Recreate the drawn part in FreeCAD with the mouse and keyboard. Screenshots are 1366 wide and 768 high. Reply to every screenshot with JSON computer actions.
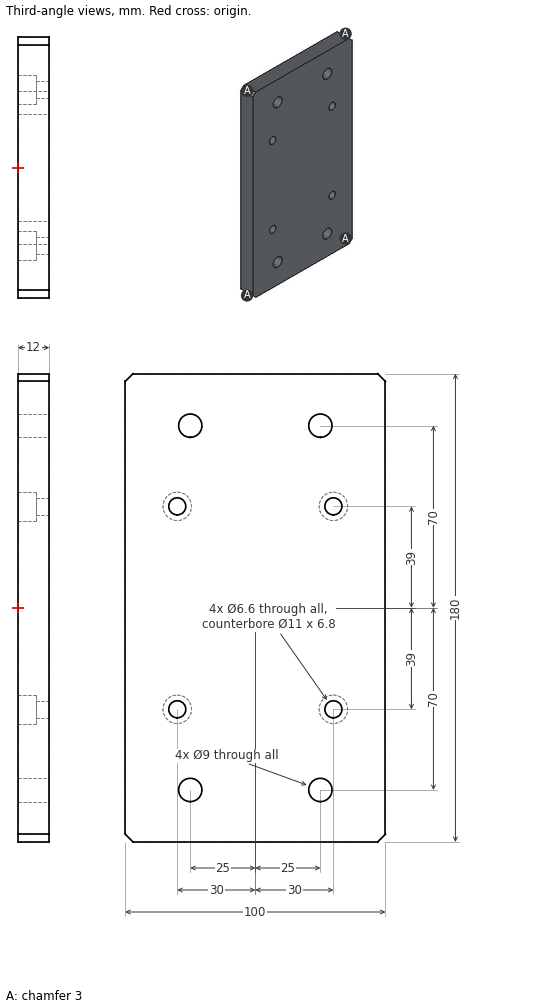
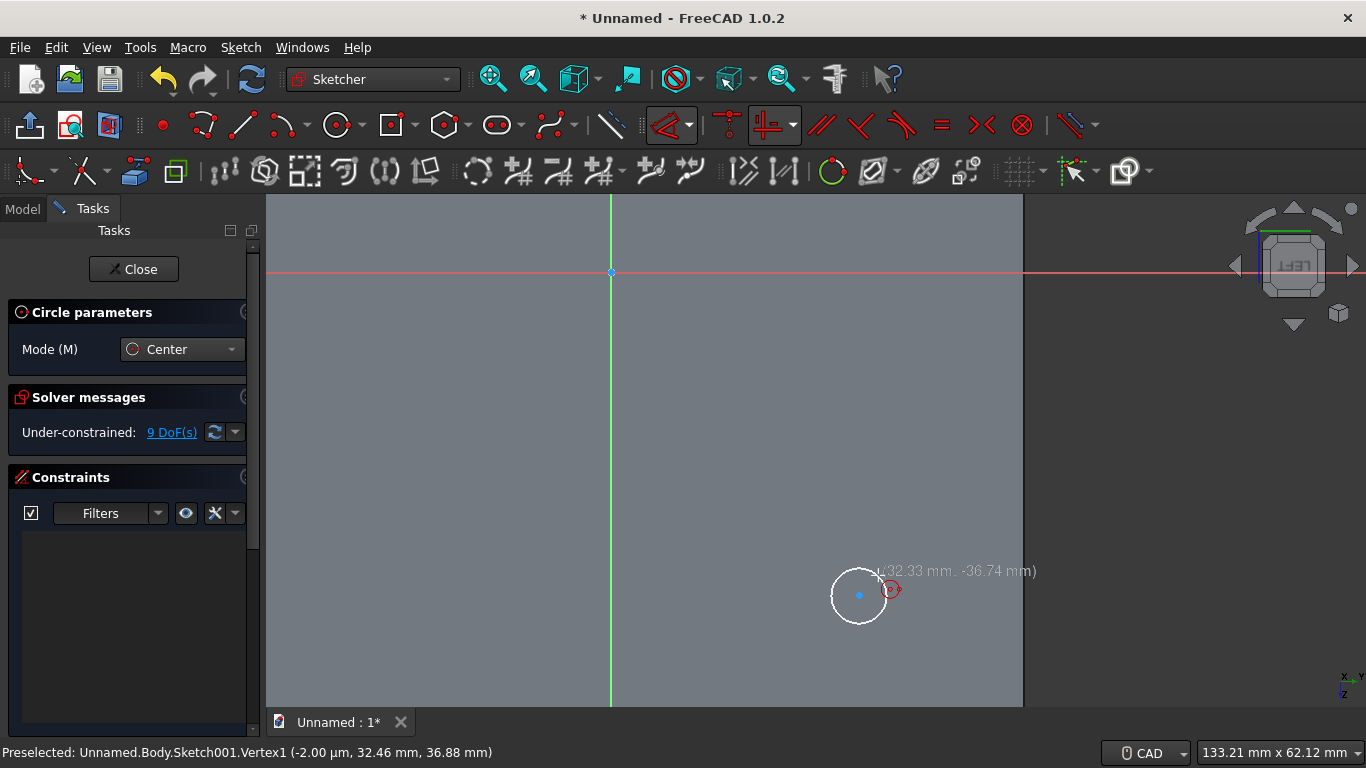
{"action": "left_click", "coordinate": [363, 595]}
{"action": "left_click", "coordinate": [383, 575]}
{"action": "key", "text": "Escape"}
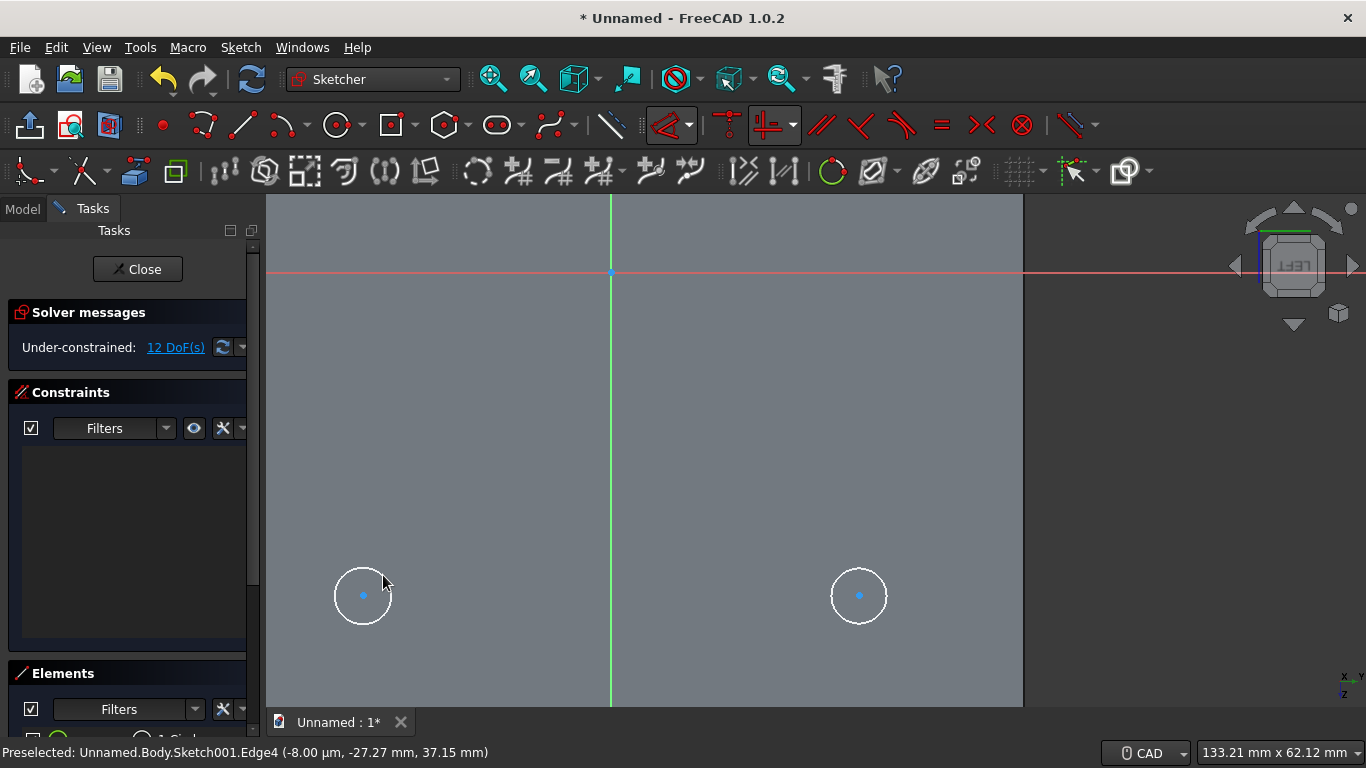
{"action": "scroll", "coordinate": [859, 596], "scroll_direction": "down", "scroll_amount": 4}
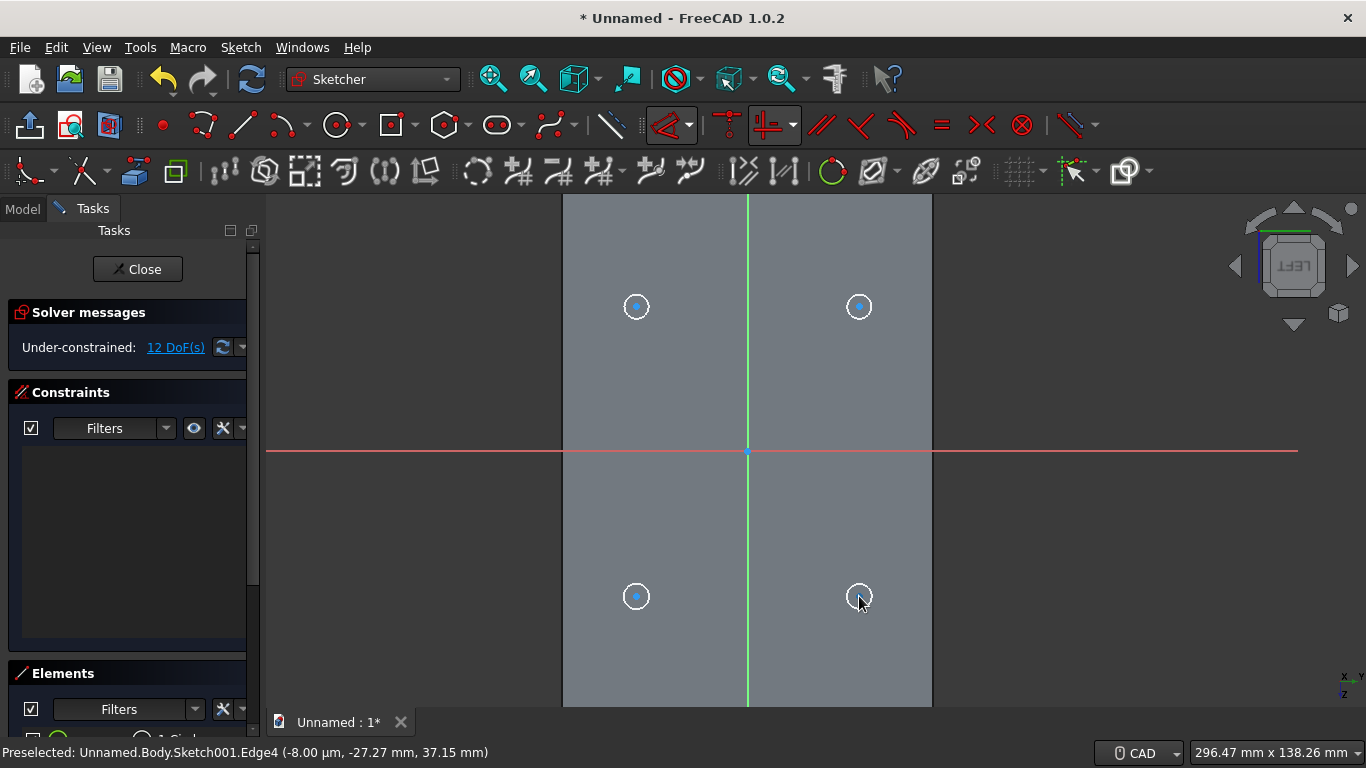
{"action": "left_click", "coordinate": [868, 298]}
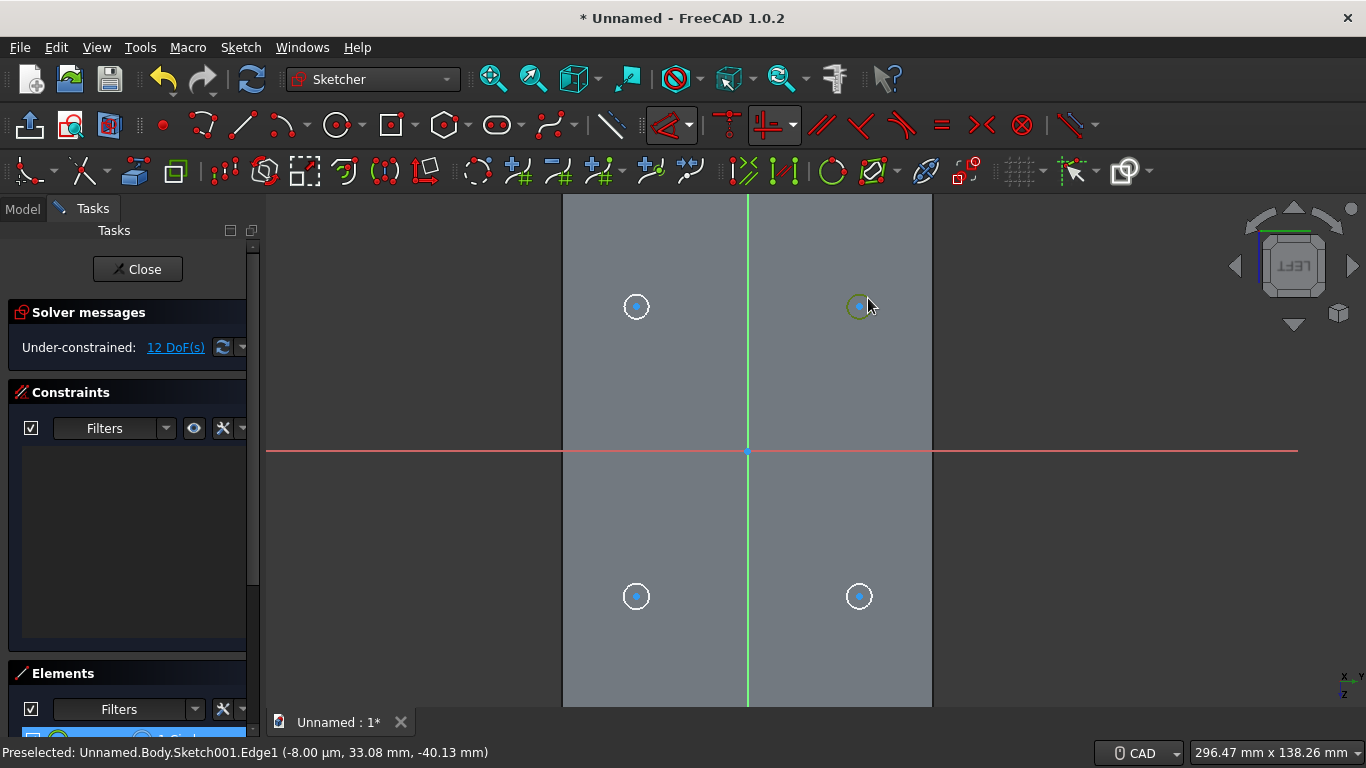
{"action": "left_click", "coordinate": [645, 298]}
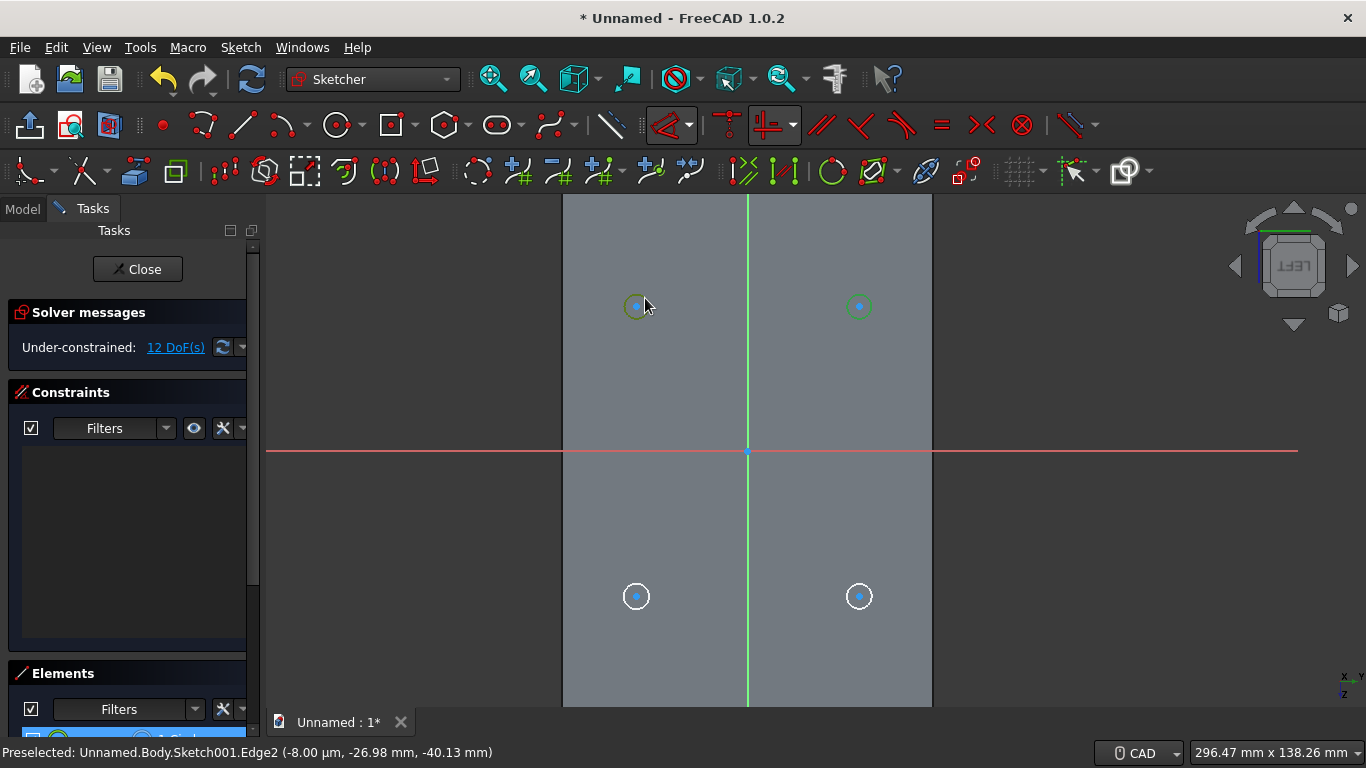
{"action": "left_click", "coordinate": [868, 588]}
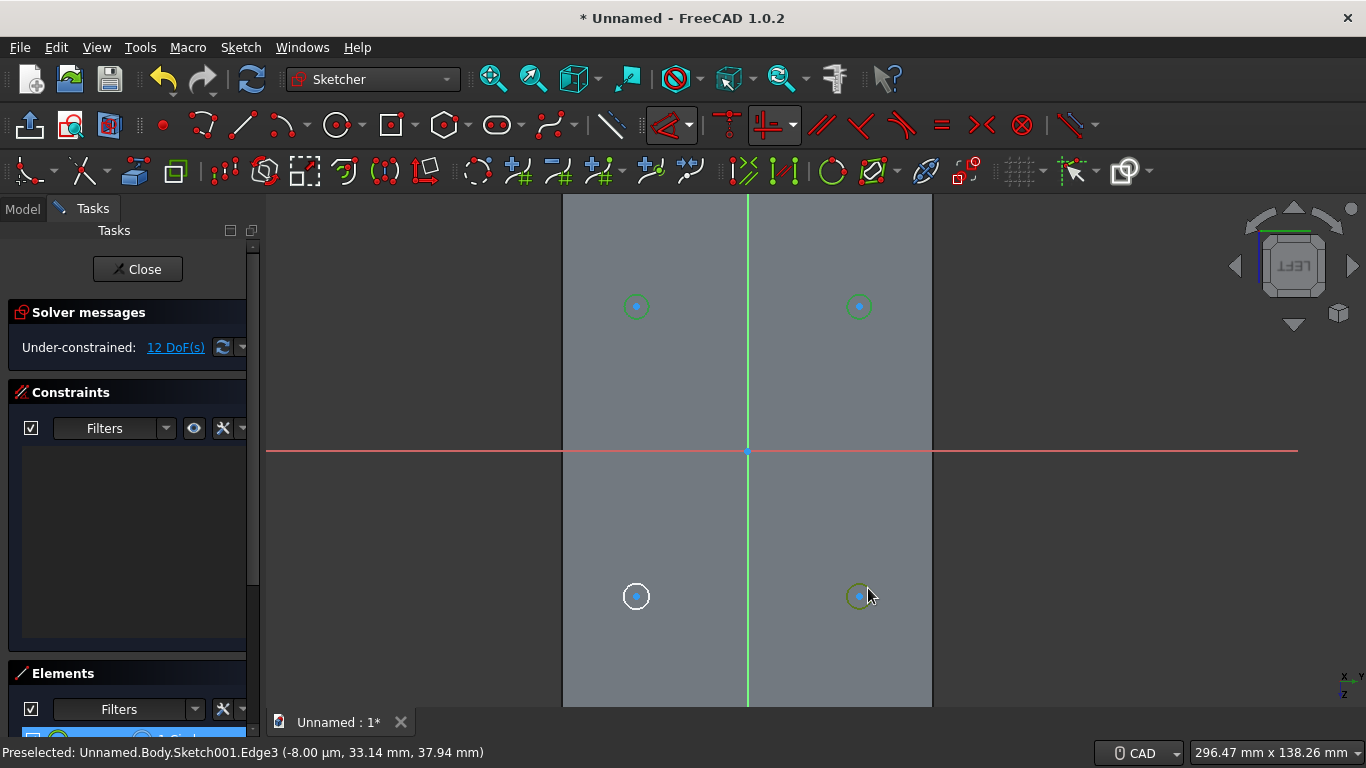
{"action": "left_click", "coordinate": [645, 587]}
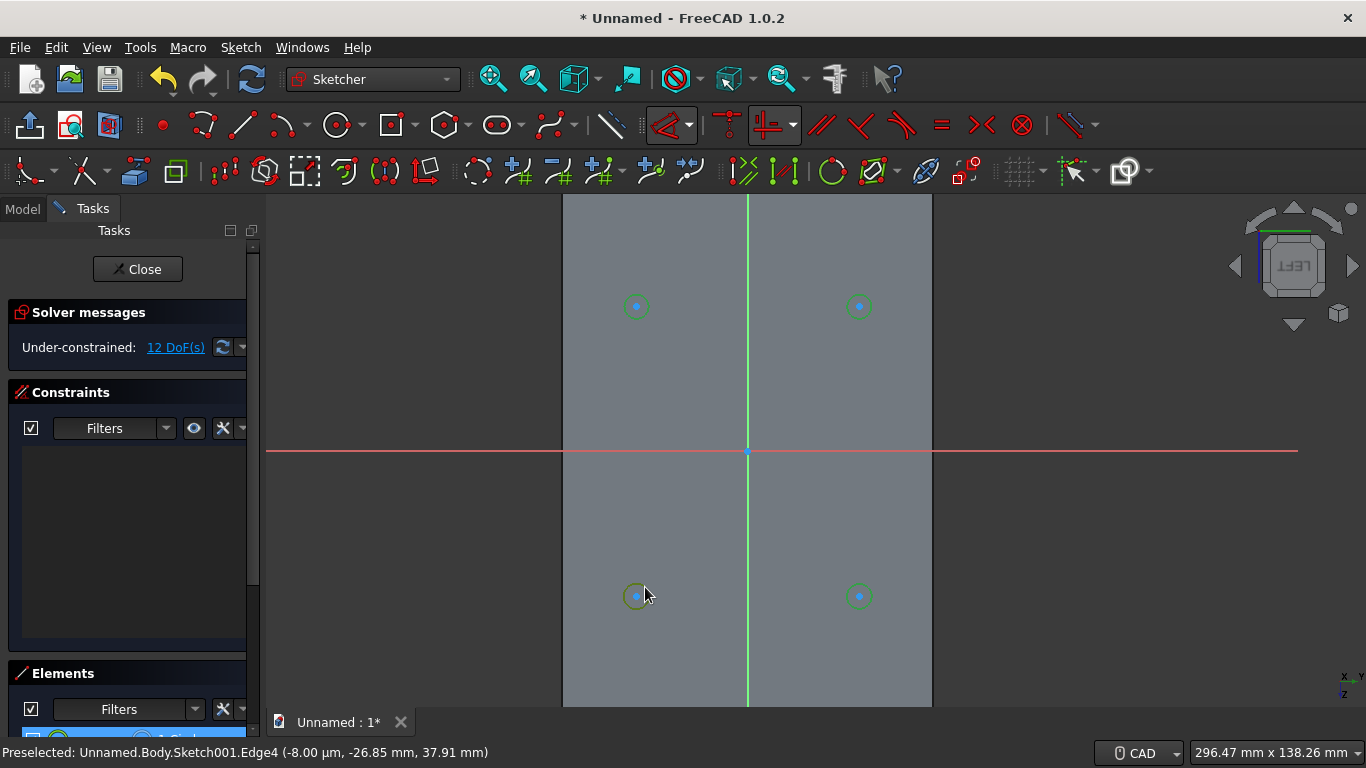
{"action": "left_click", "coordinate": [942, 126]}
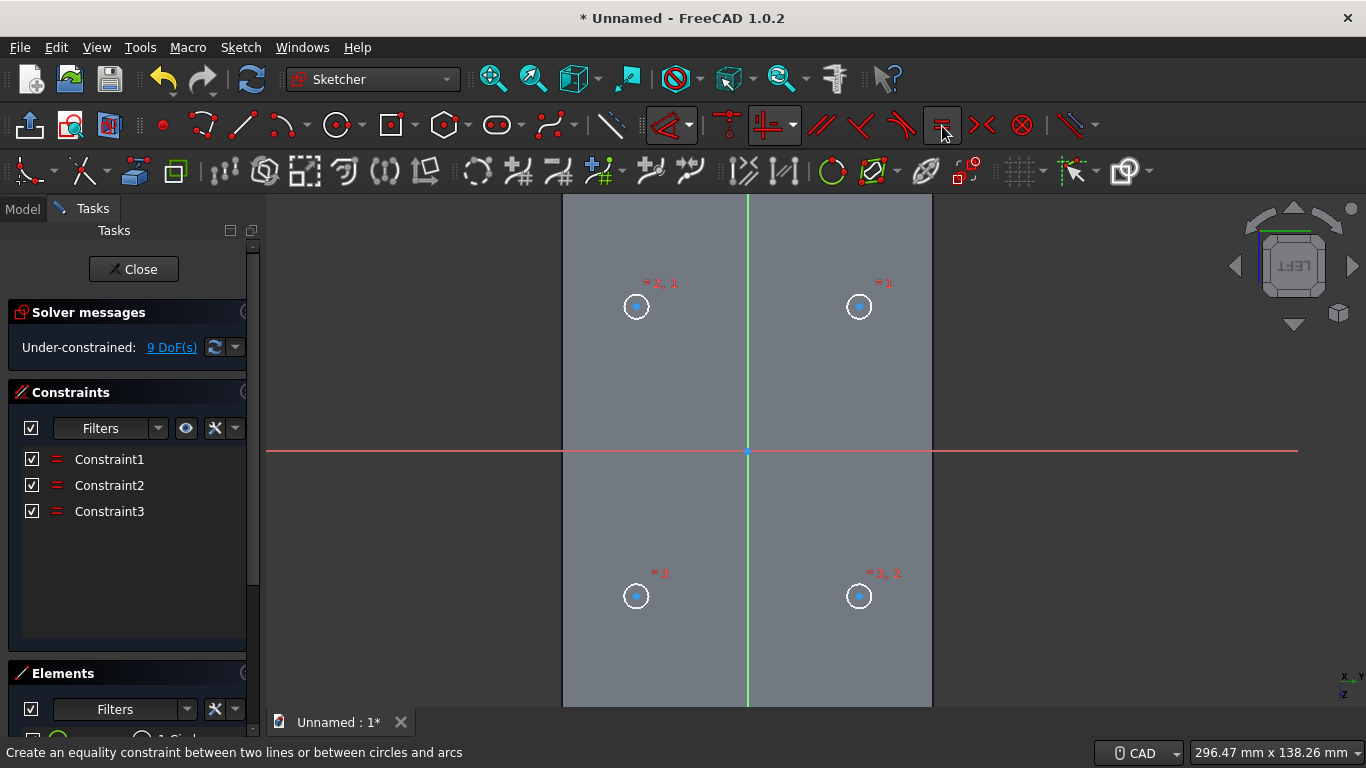
{"action": "left_click", "coordinate": [859, 307]}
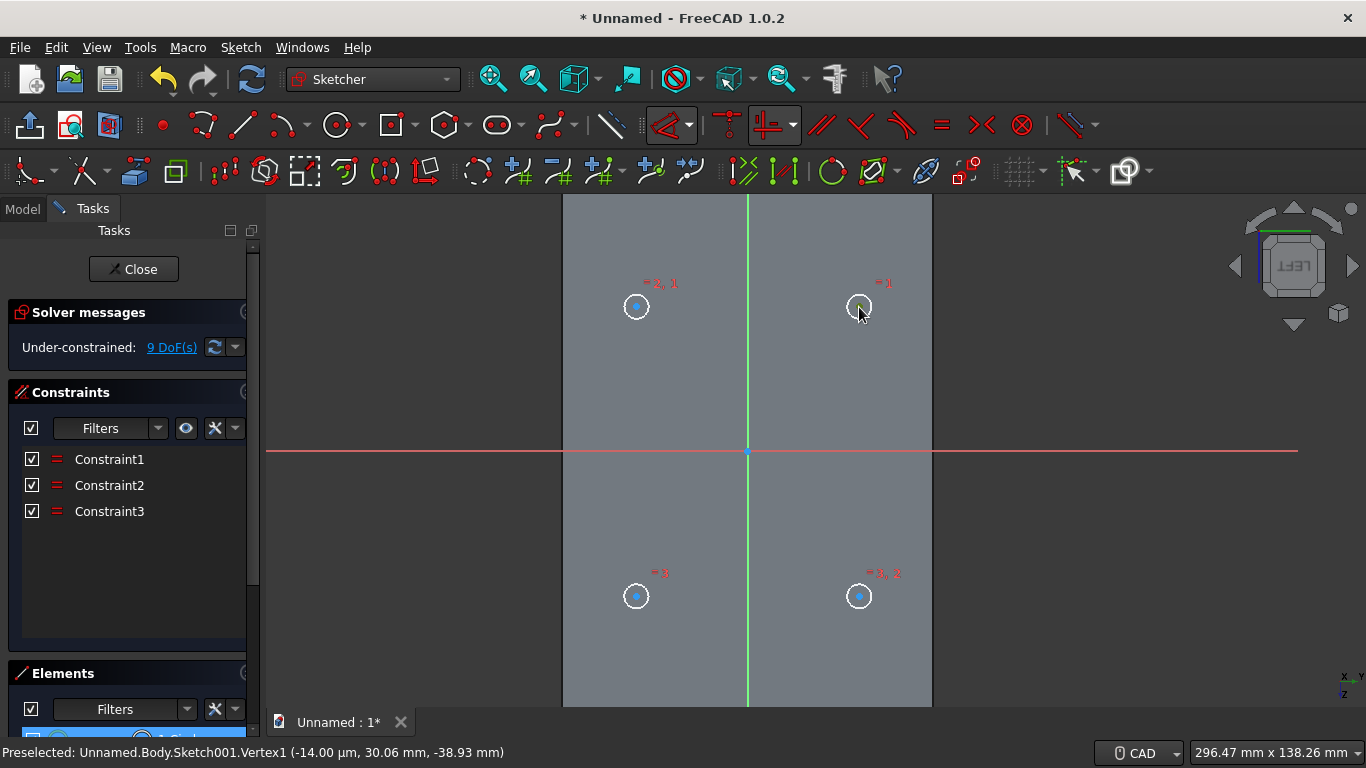
{"action": "left_click", "coordinate": [637, 307]}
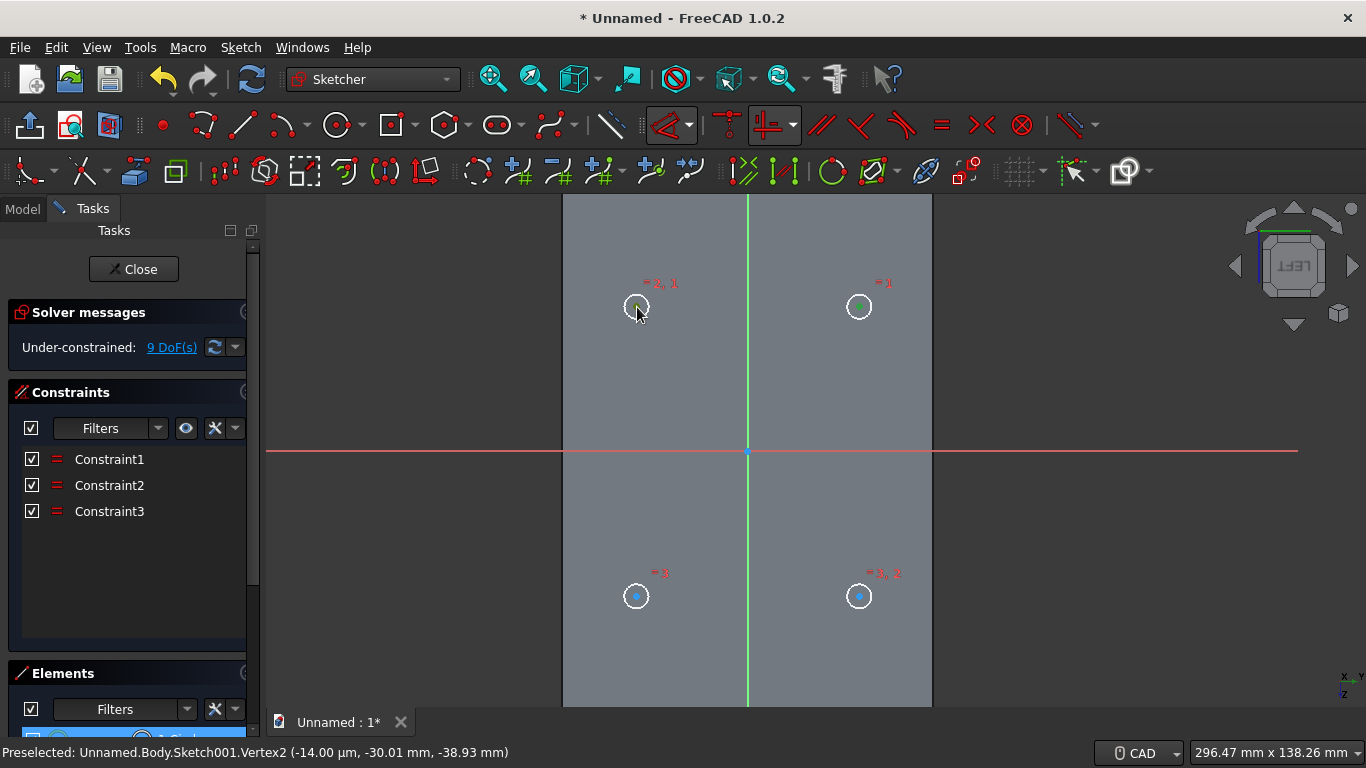
{"action": "key", "text": "h"}